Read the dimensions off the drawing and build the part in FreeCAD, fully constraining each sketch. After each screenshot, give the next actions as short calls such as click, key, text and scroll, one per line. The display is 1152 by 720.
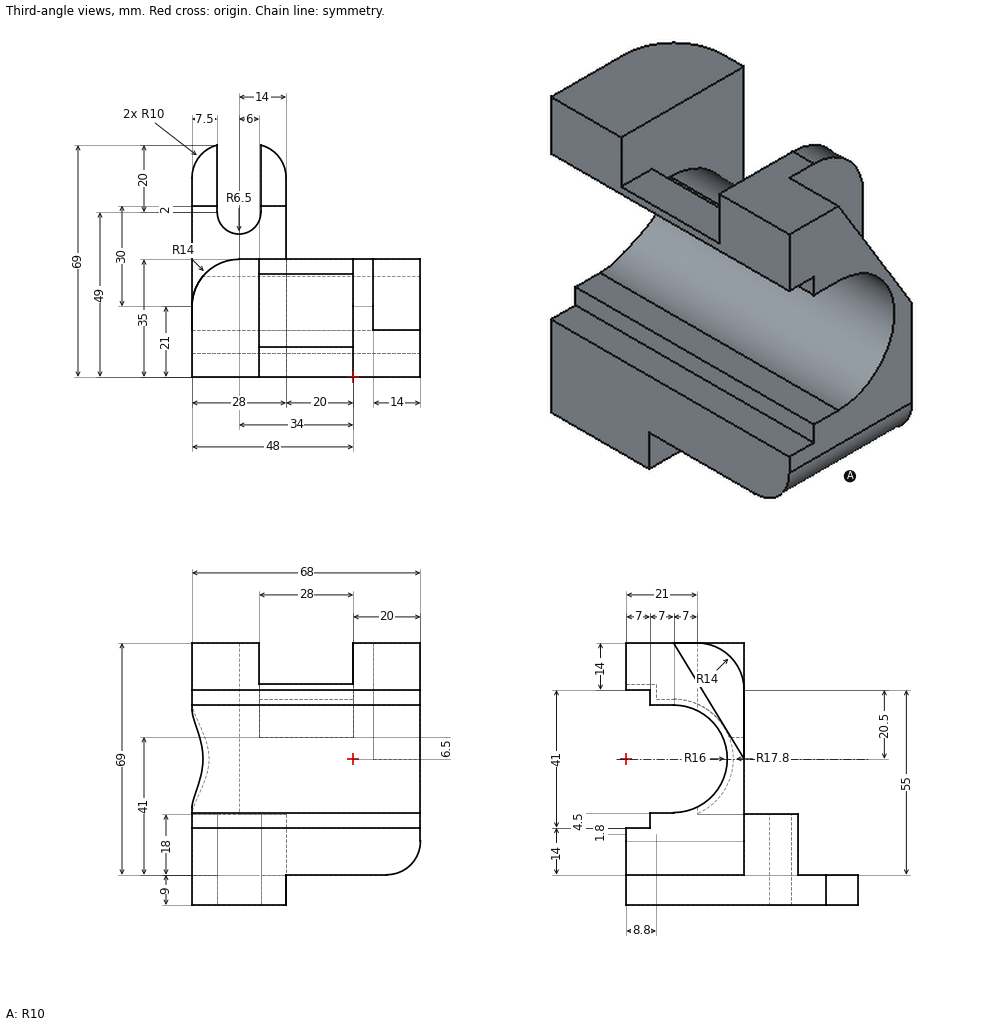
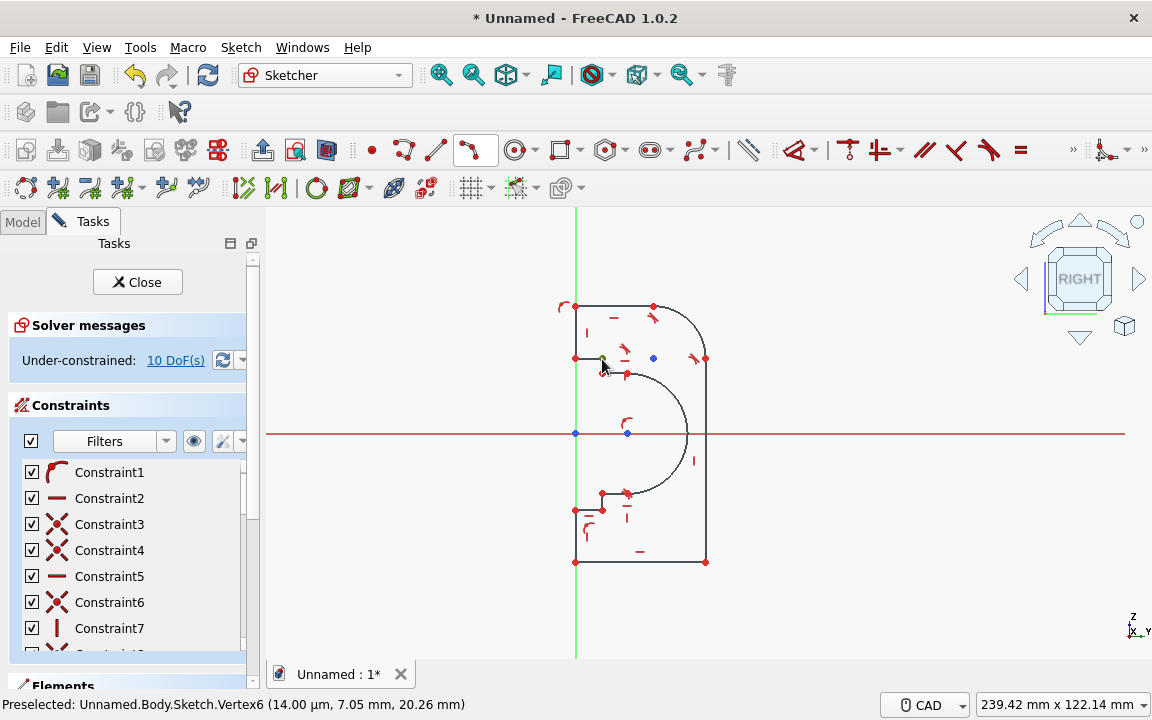
click(602, 510)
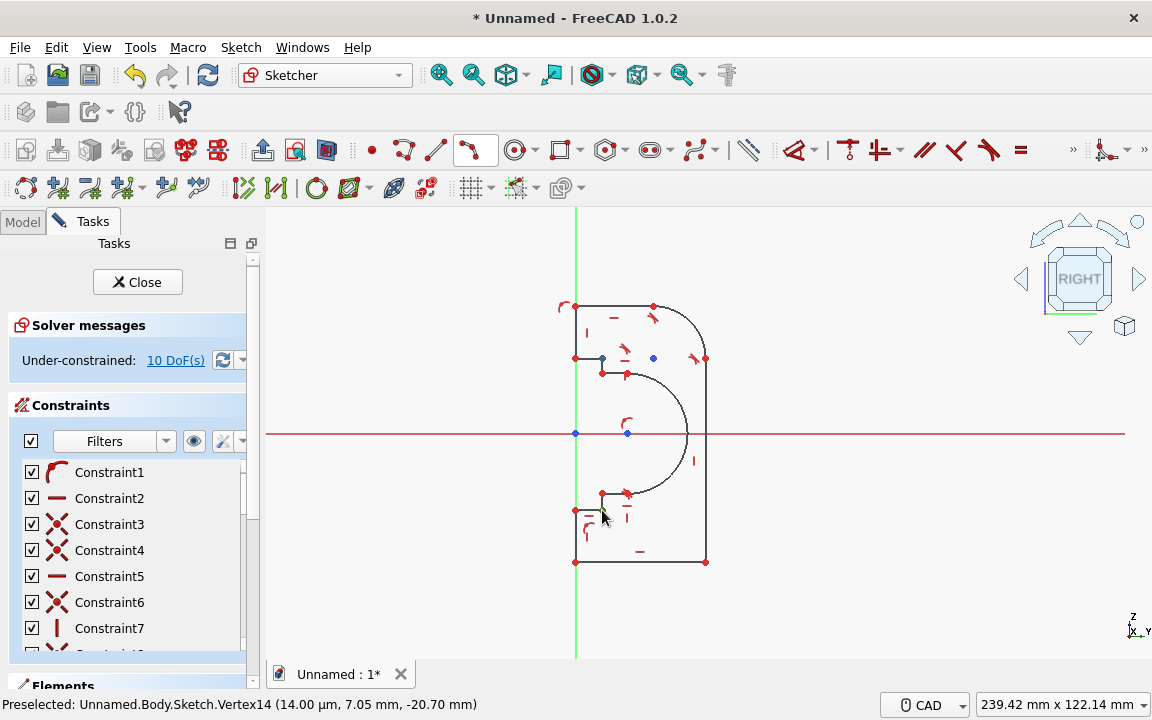
click(344, 434)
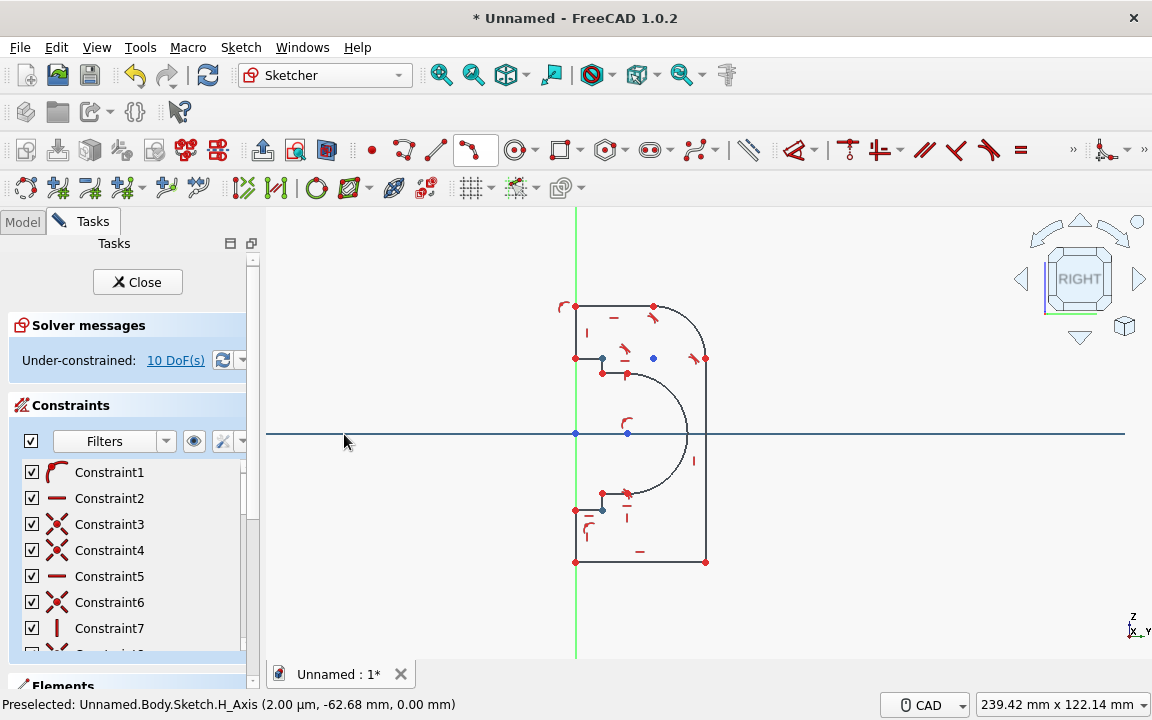
key(s)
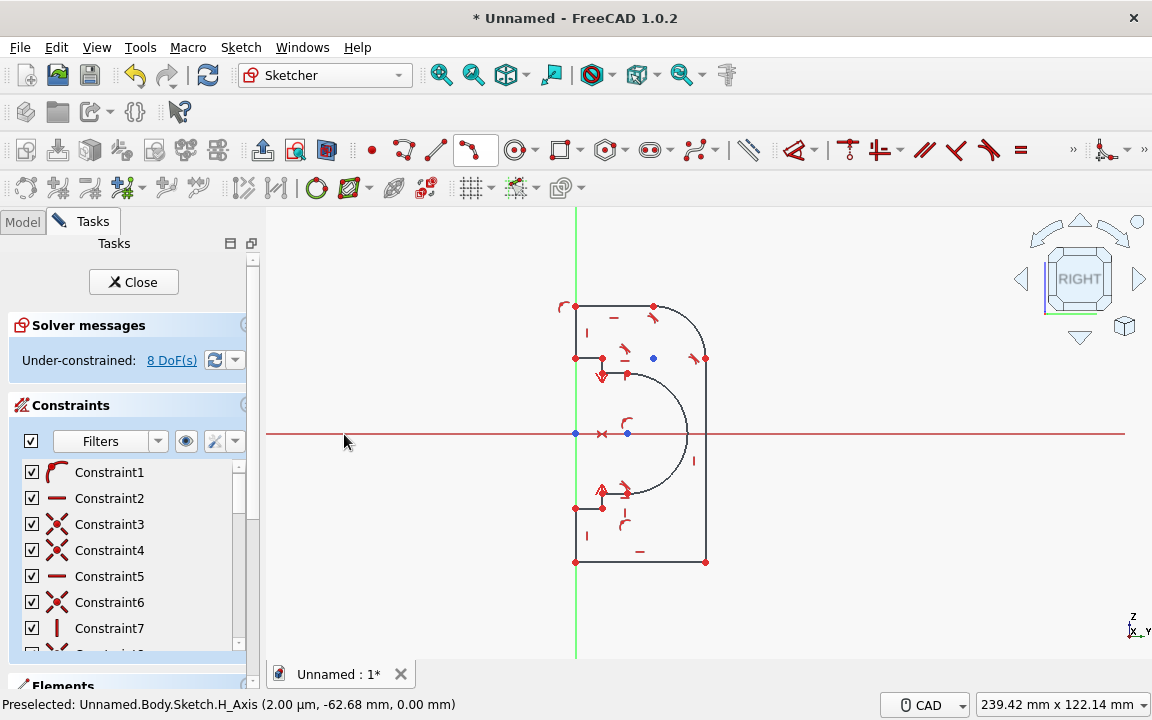
click(794, 150)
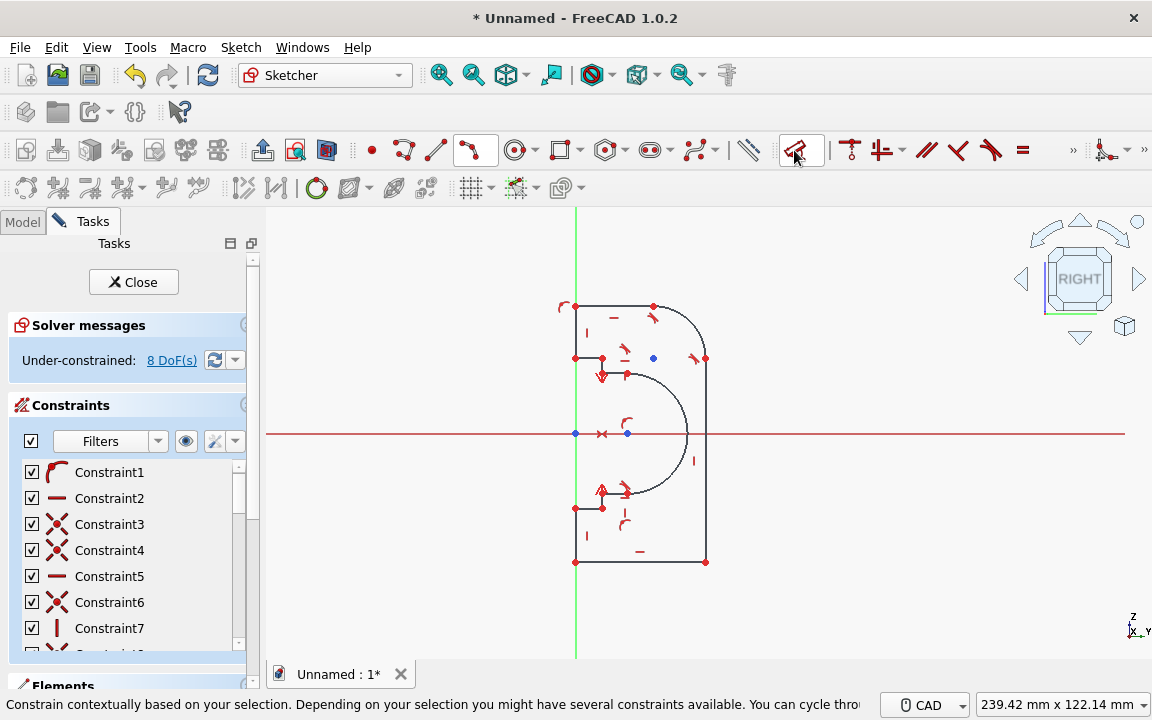
click(676, 469)
click(667, 517)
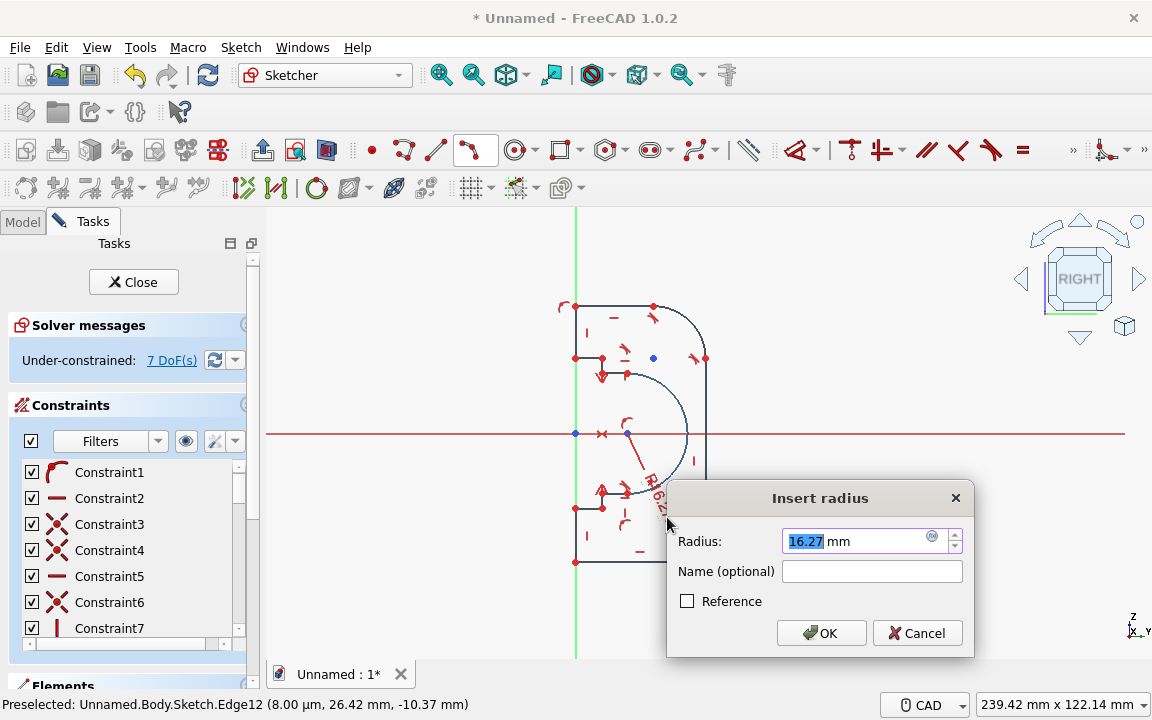
text(16)
key(Return)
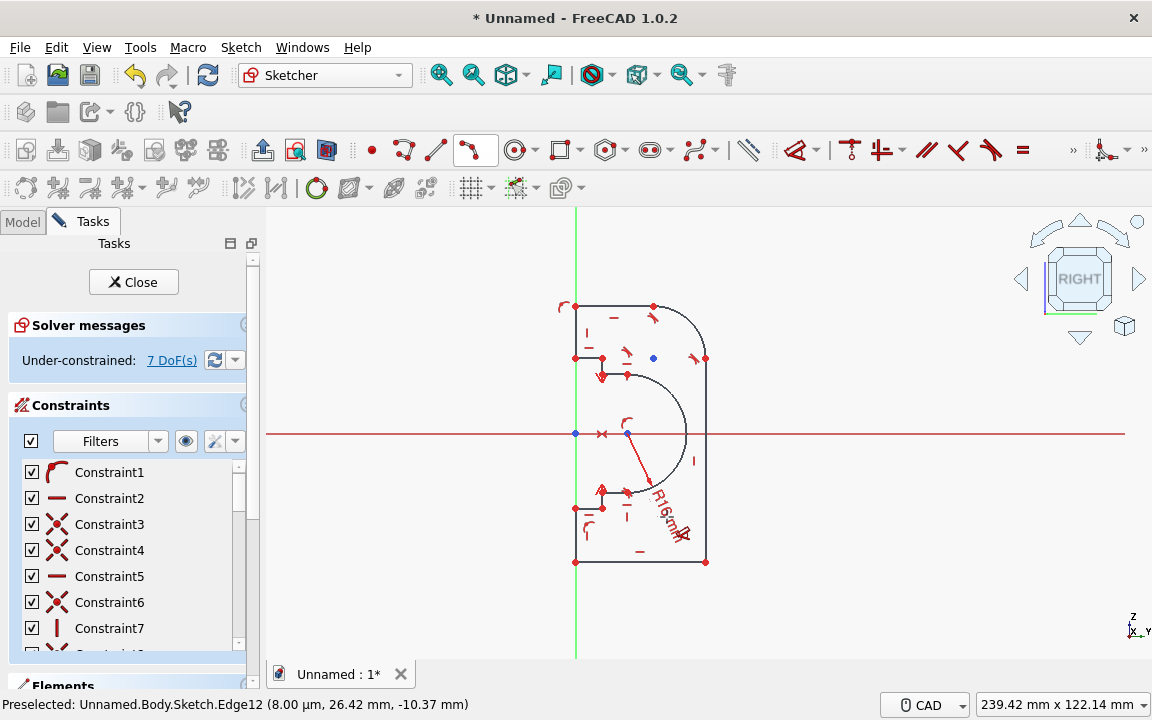
click(700, 335)
click(729, 321)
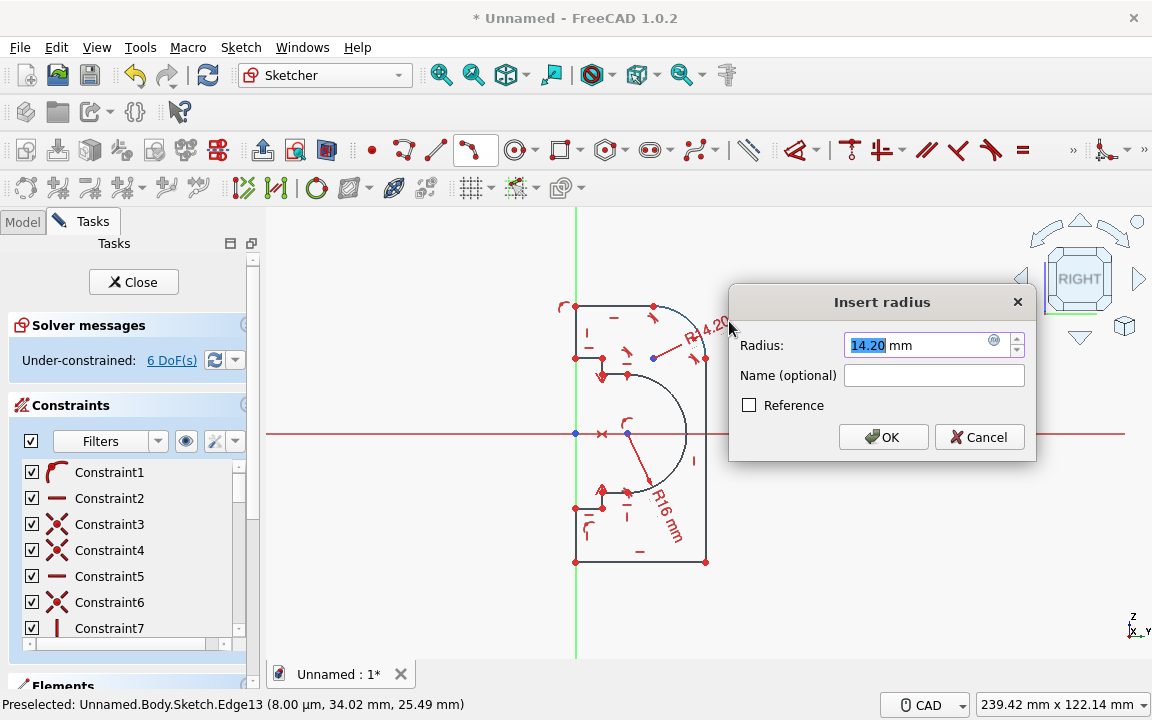
text(14)
key(Return)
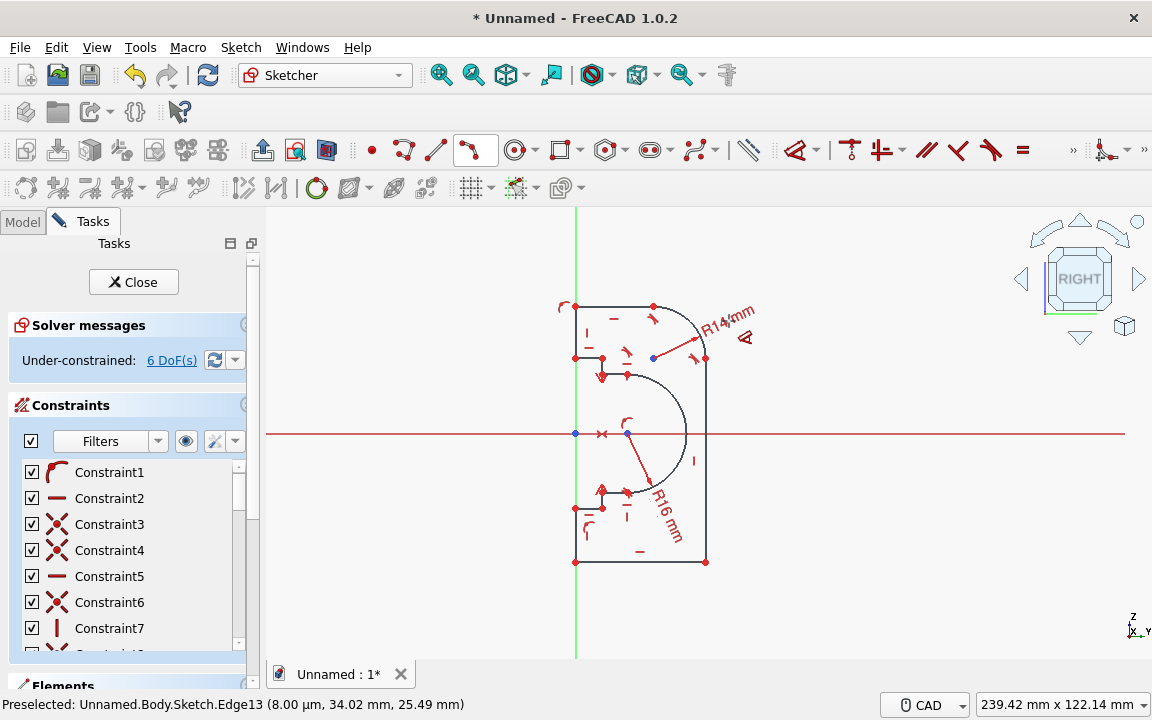
scroll(586, 358, up, 3)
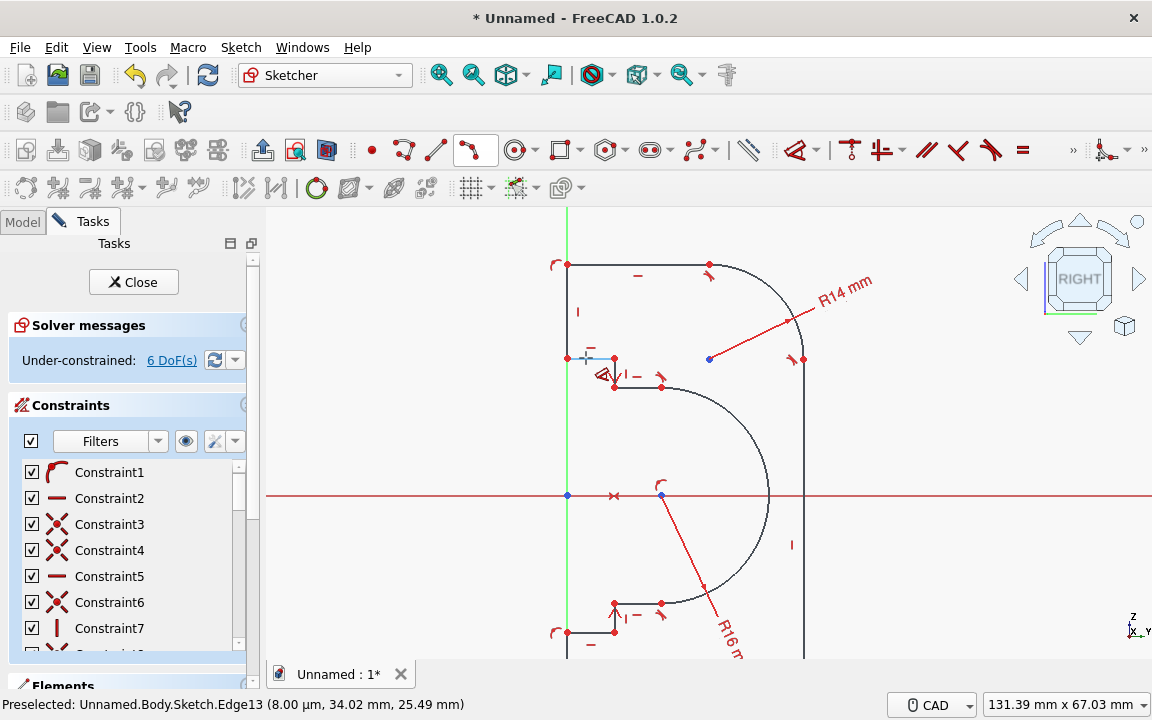
click(586, 359)
click(591, 325)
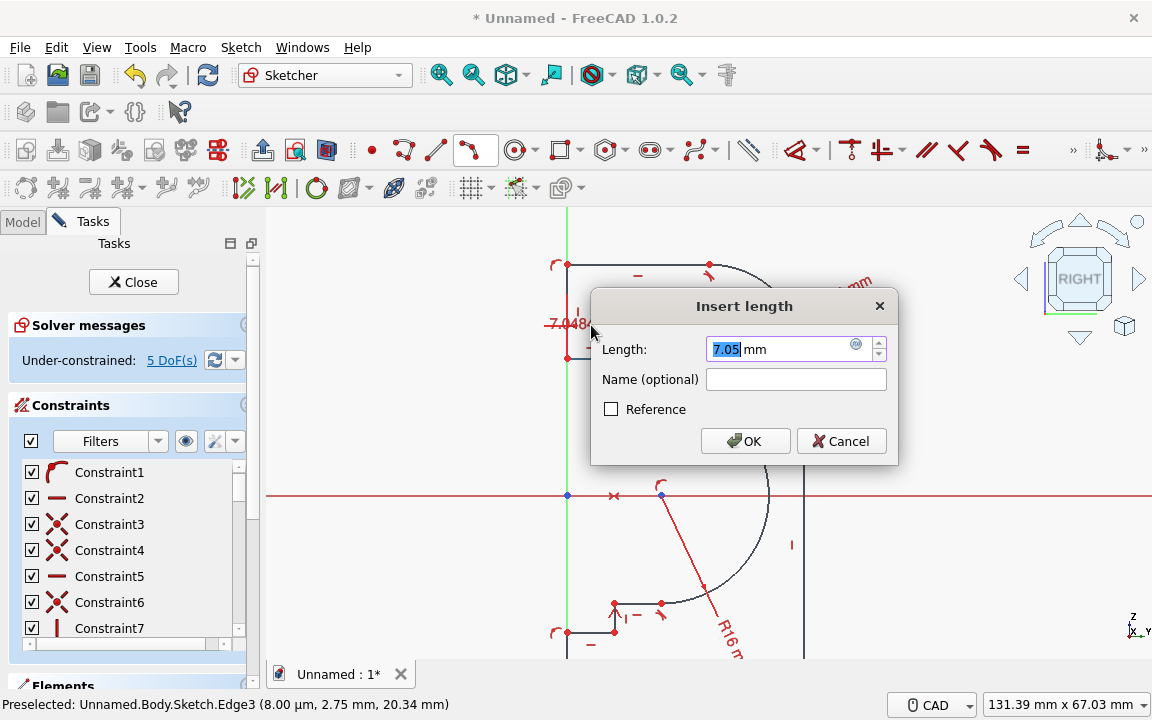
text(7)
key(Return)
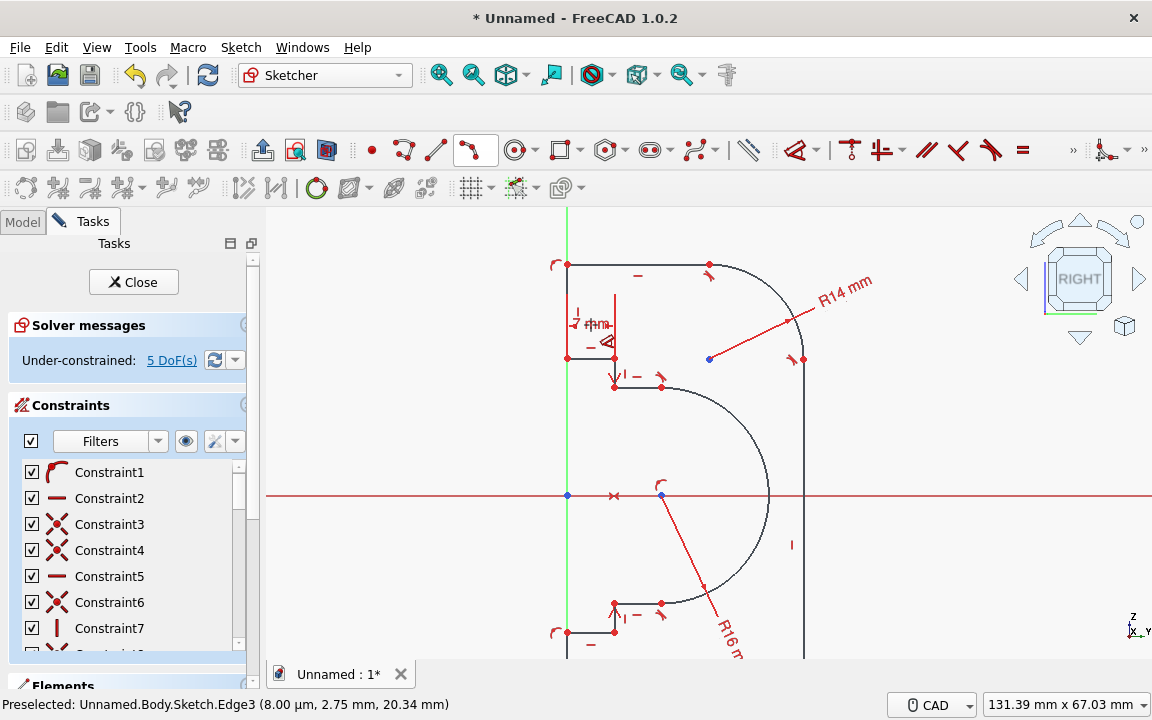
click(629, 388)
click(638, 354)